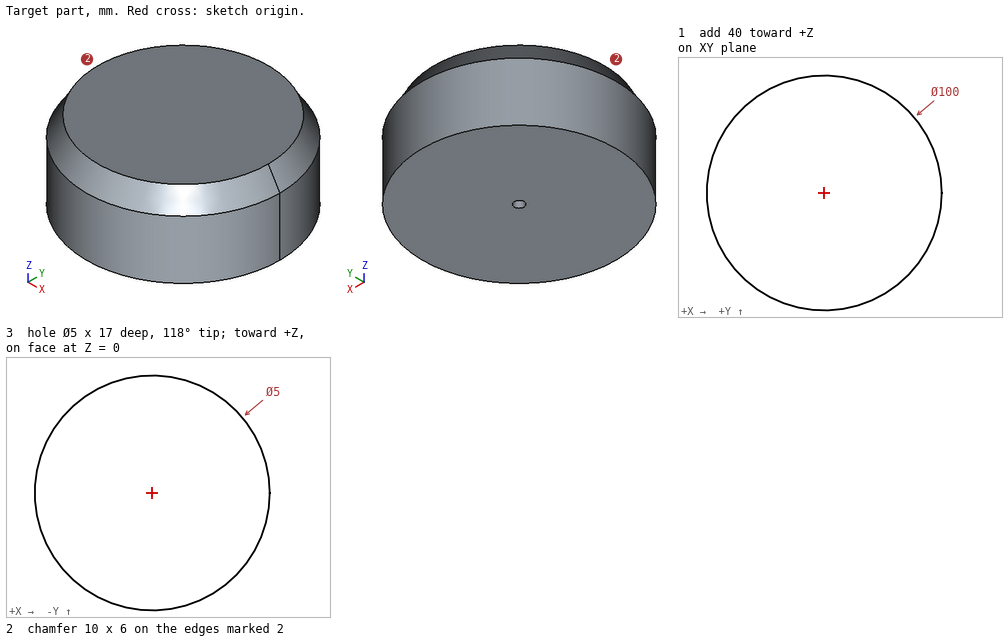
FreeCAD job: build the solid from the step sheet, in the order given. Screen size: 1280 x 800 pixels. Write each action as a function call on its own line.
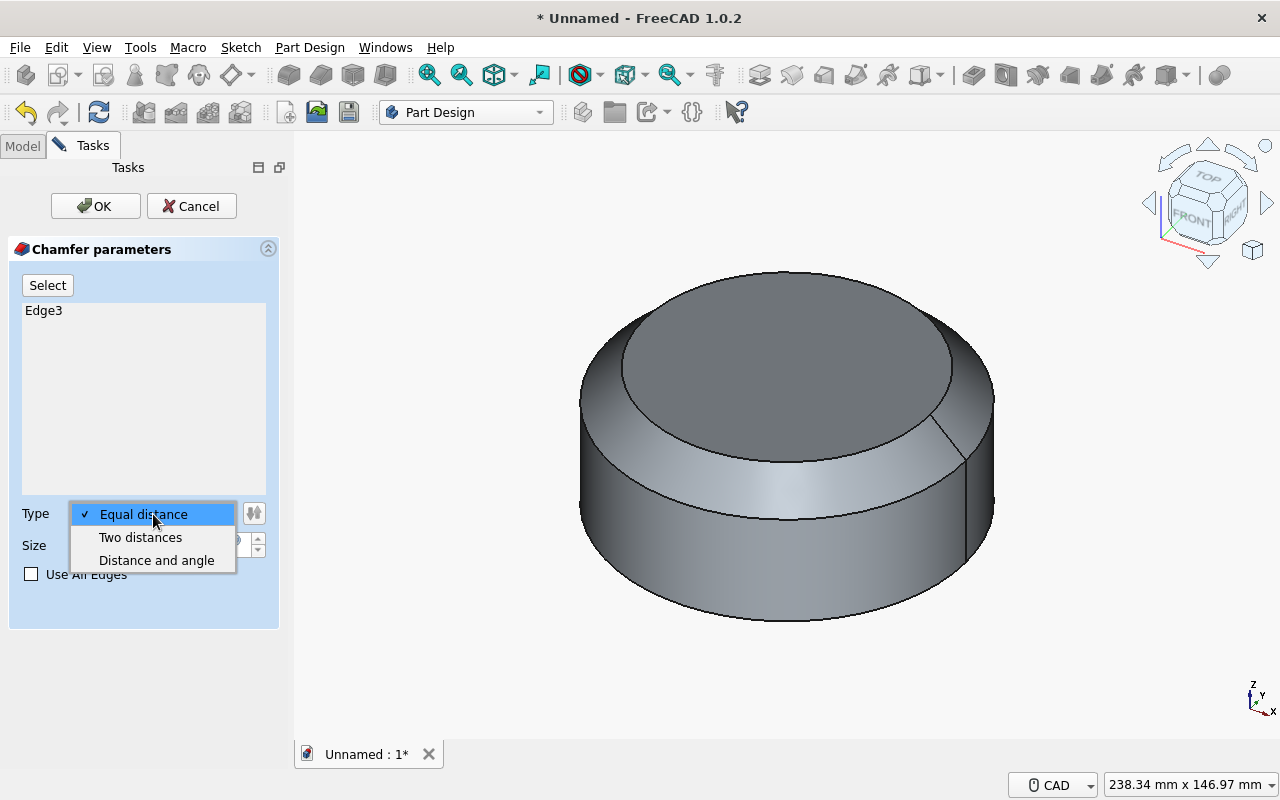
click(152, 538)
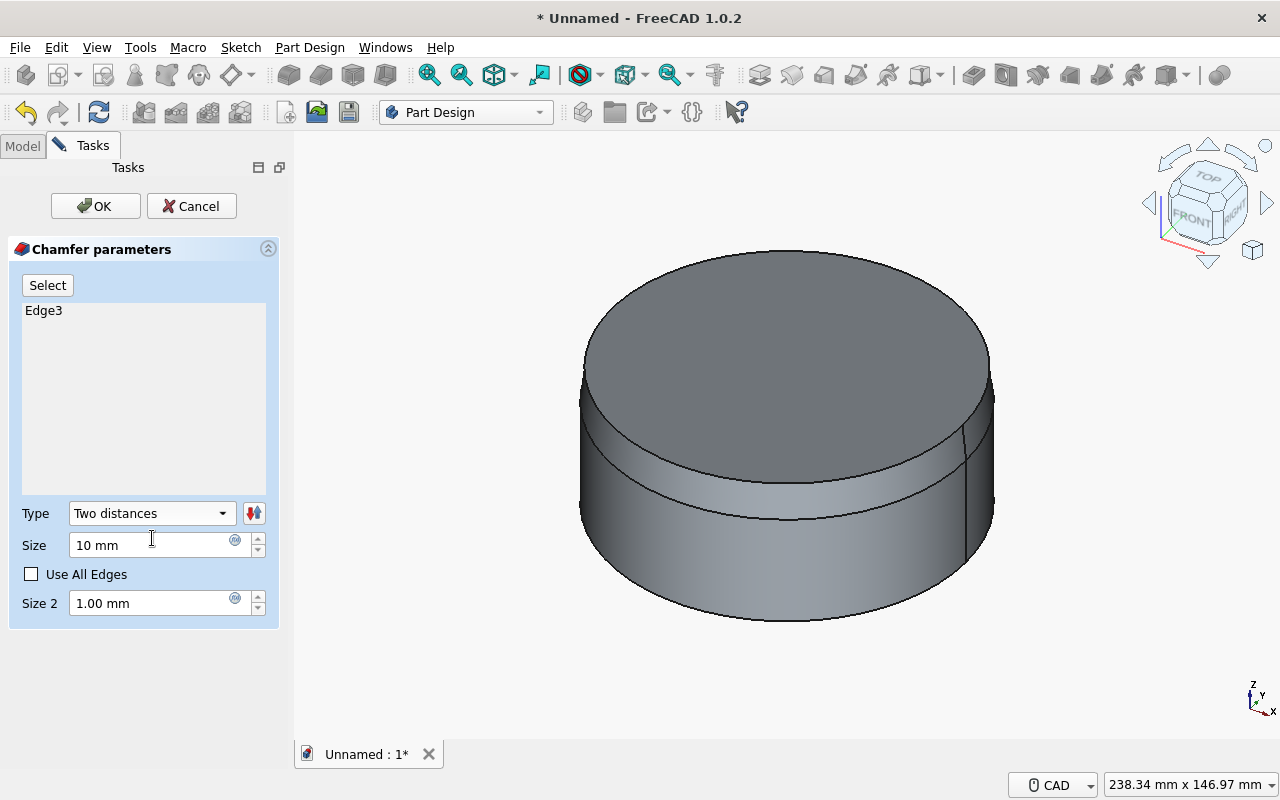
triple_click(160, 603)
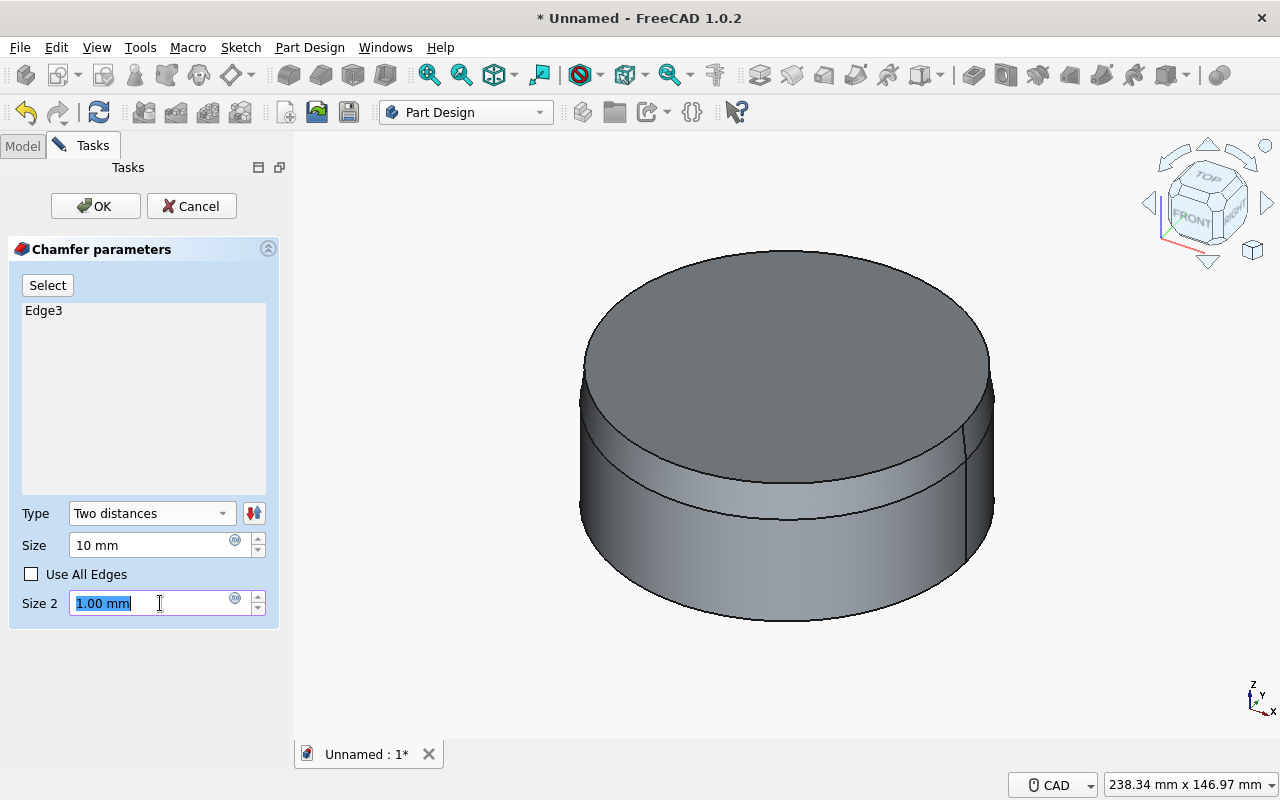
text(6)
key(Tab)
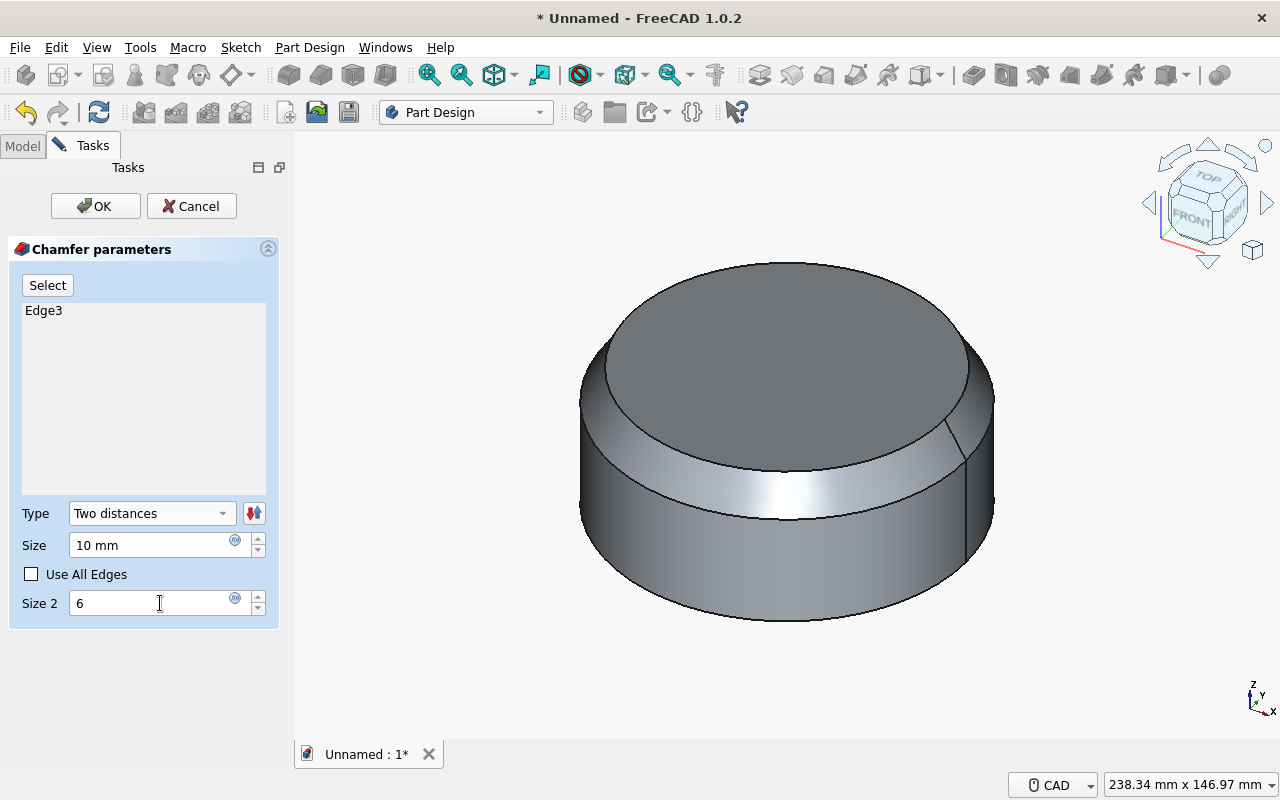
click(96, 206)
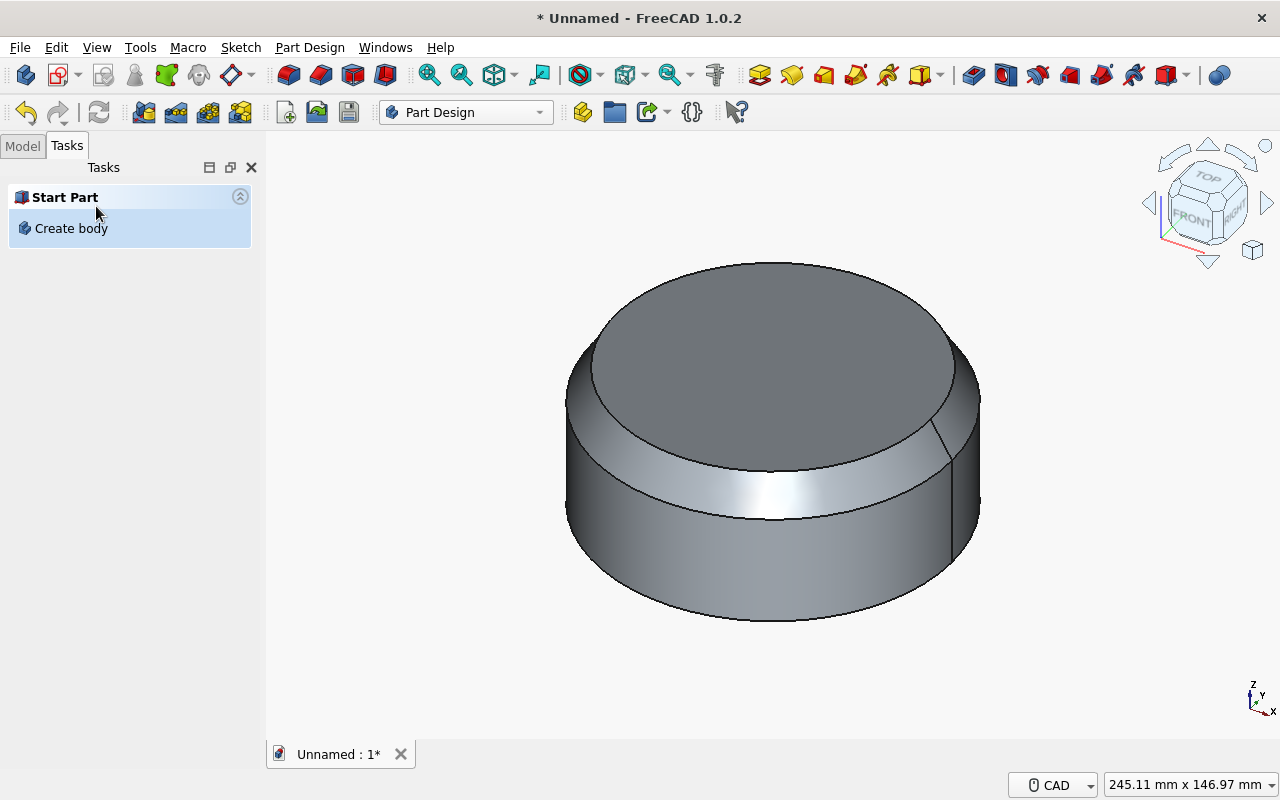
key(5)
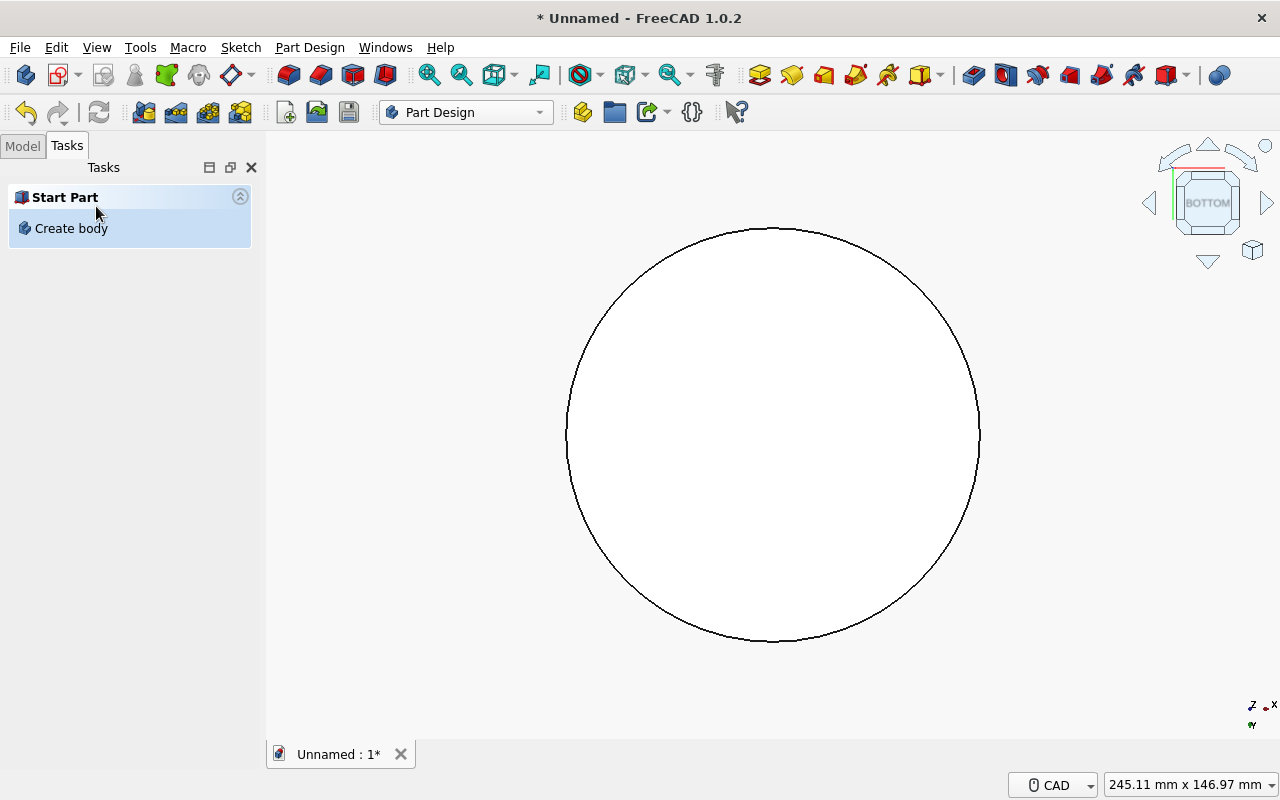
click(773, 434)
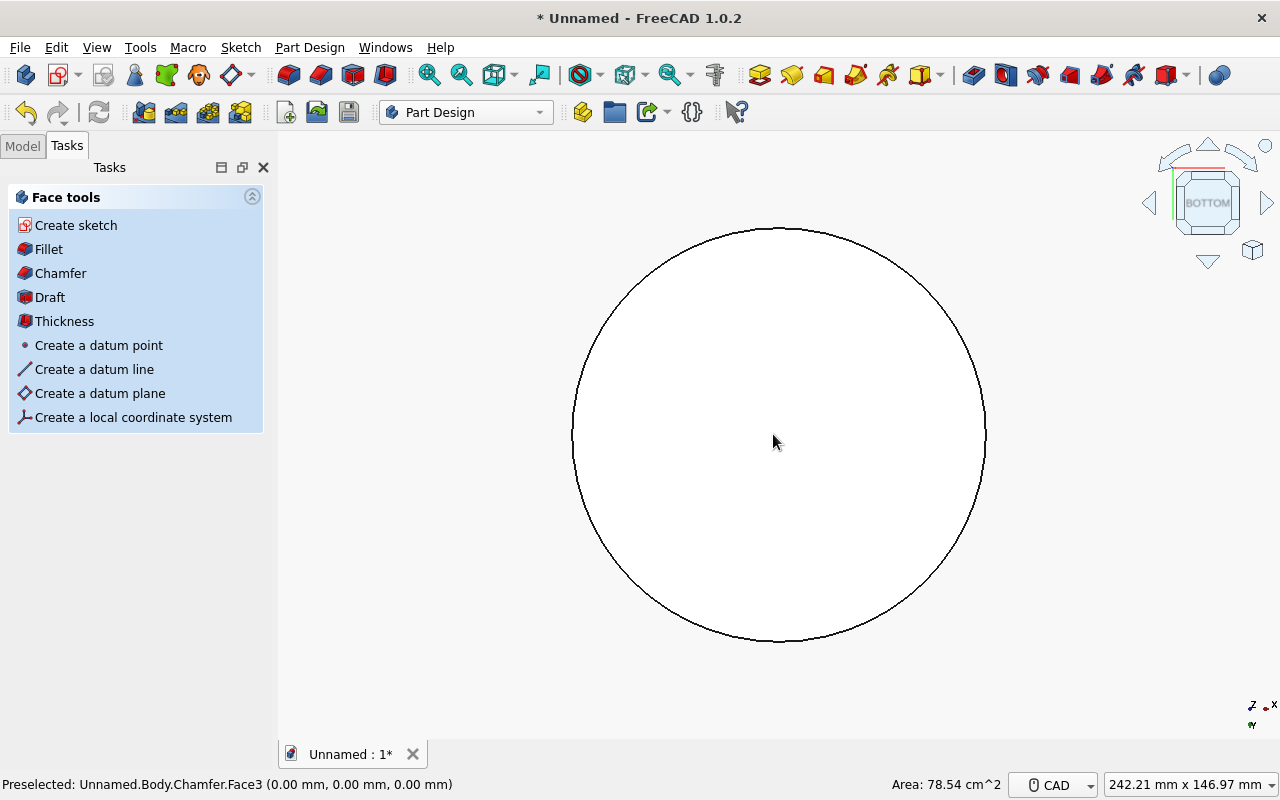
click(58, 76)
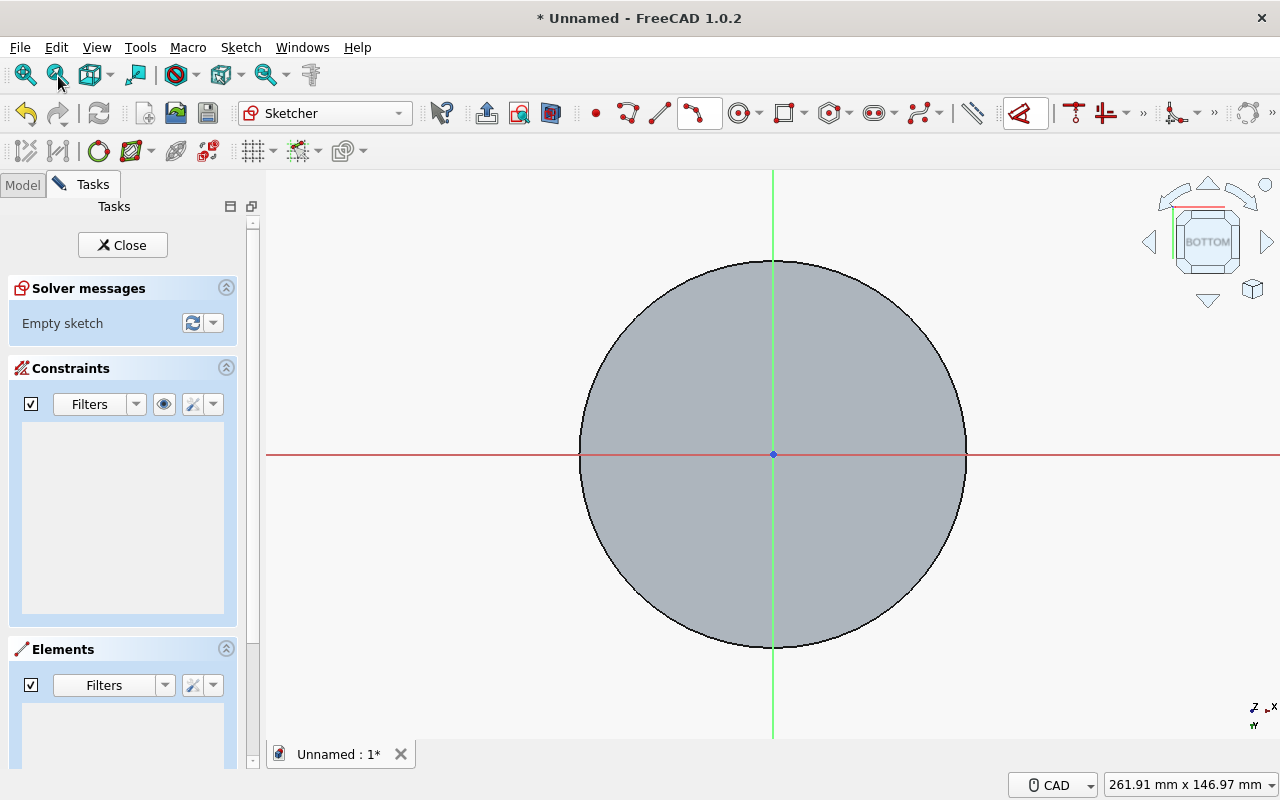
scroll(777, 455, up, 15)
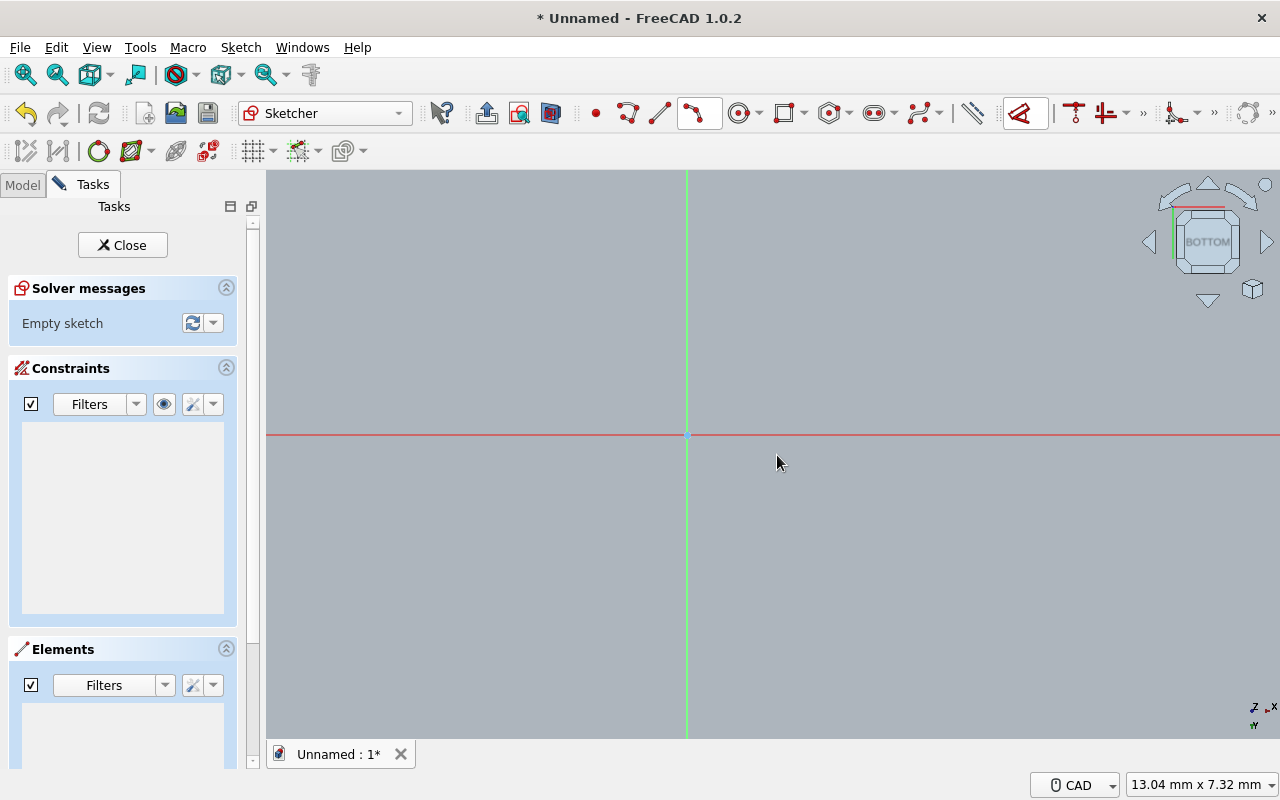
click(740, 114)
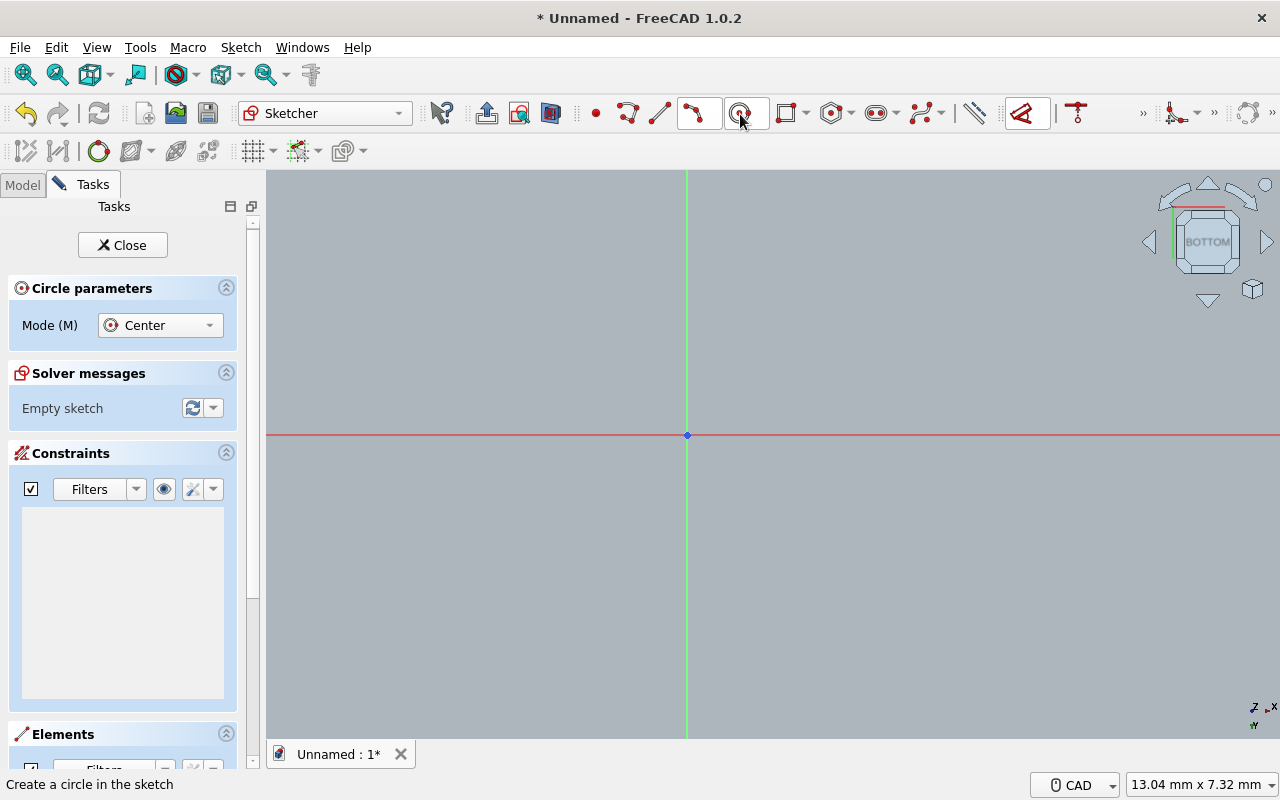
click(687, 435)
click(824, 298)
key(Escape)